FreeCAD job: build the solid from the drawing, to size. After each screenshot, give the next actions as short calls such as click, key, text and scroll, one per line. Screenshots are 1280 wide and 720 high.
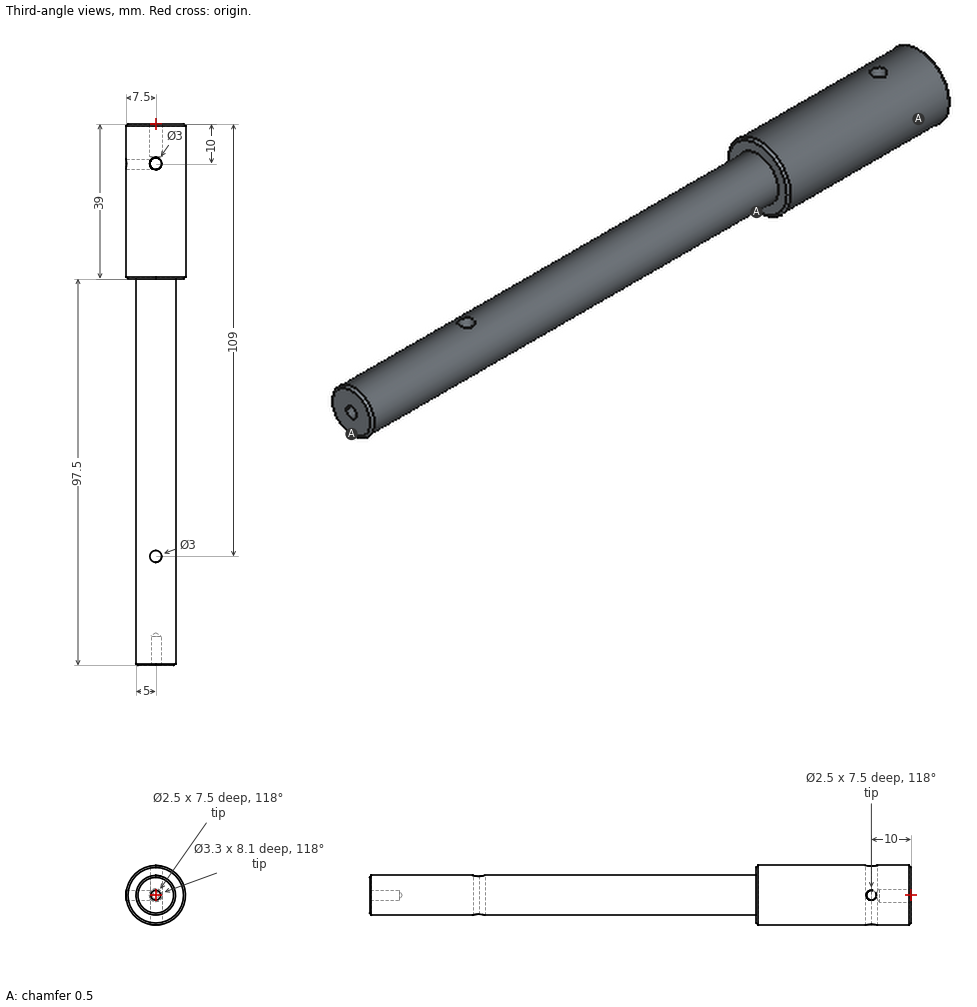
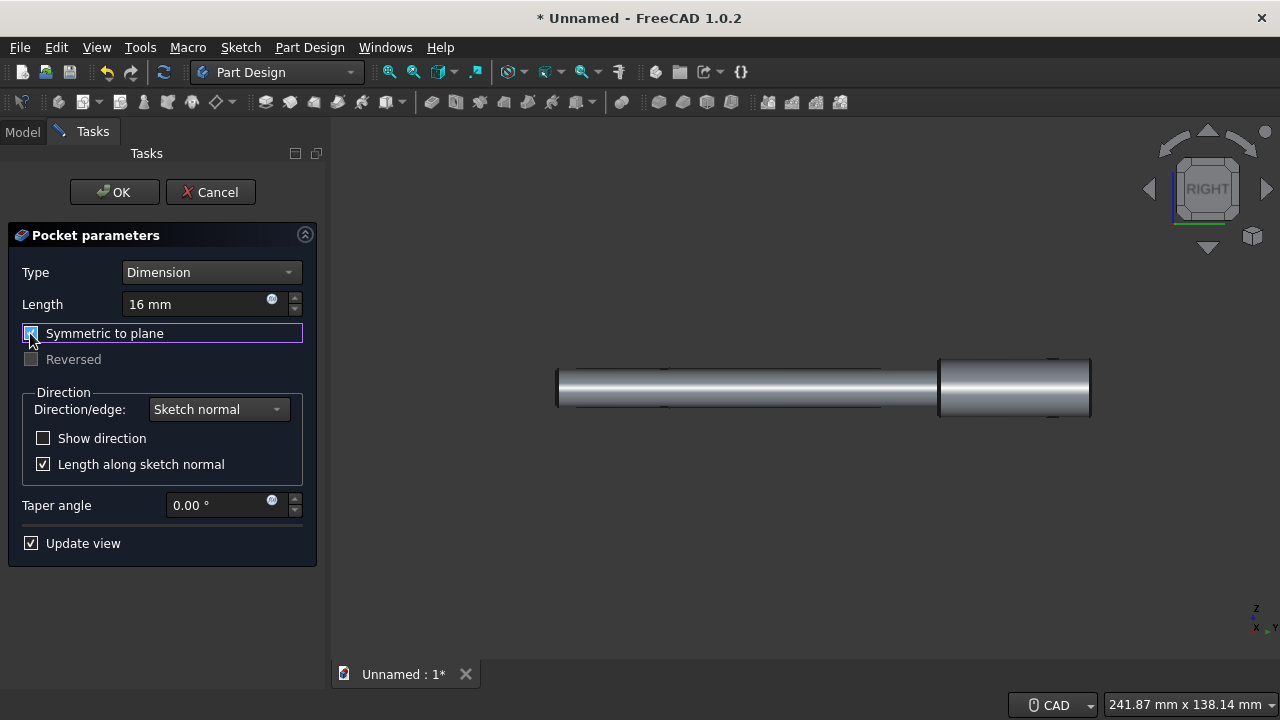
click(115, 192)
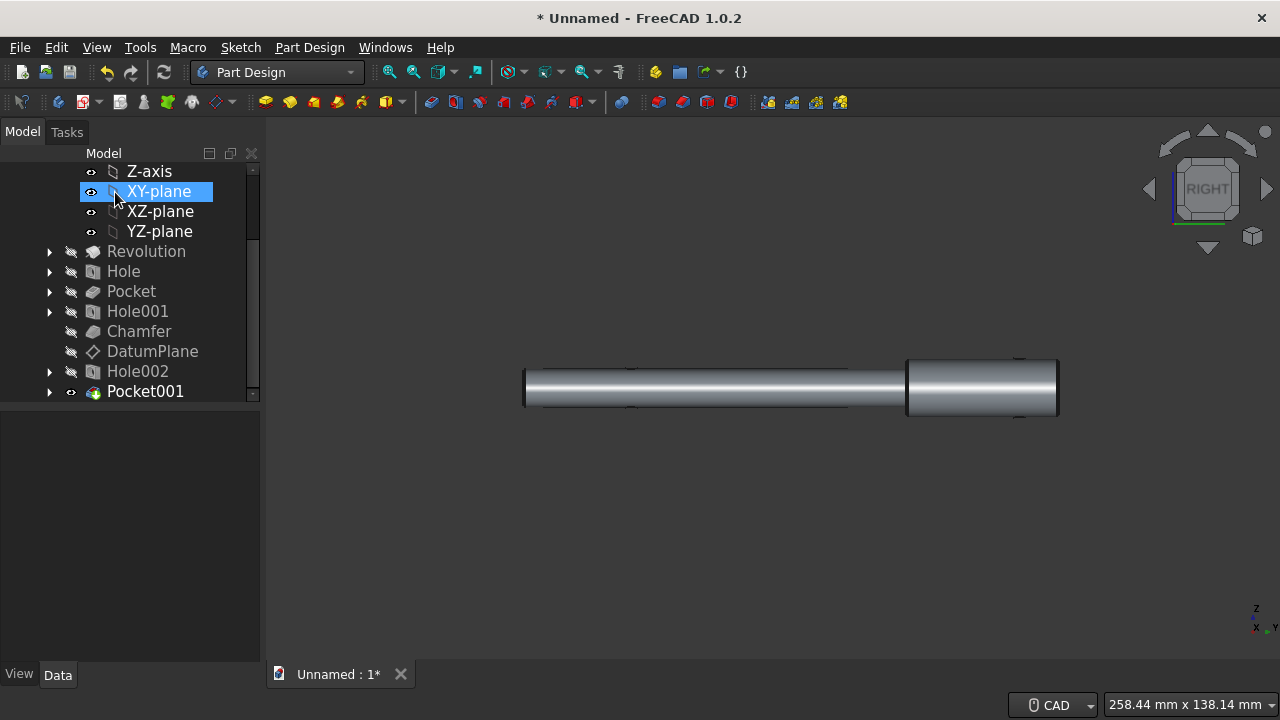
key(0)